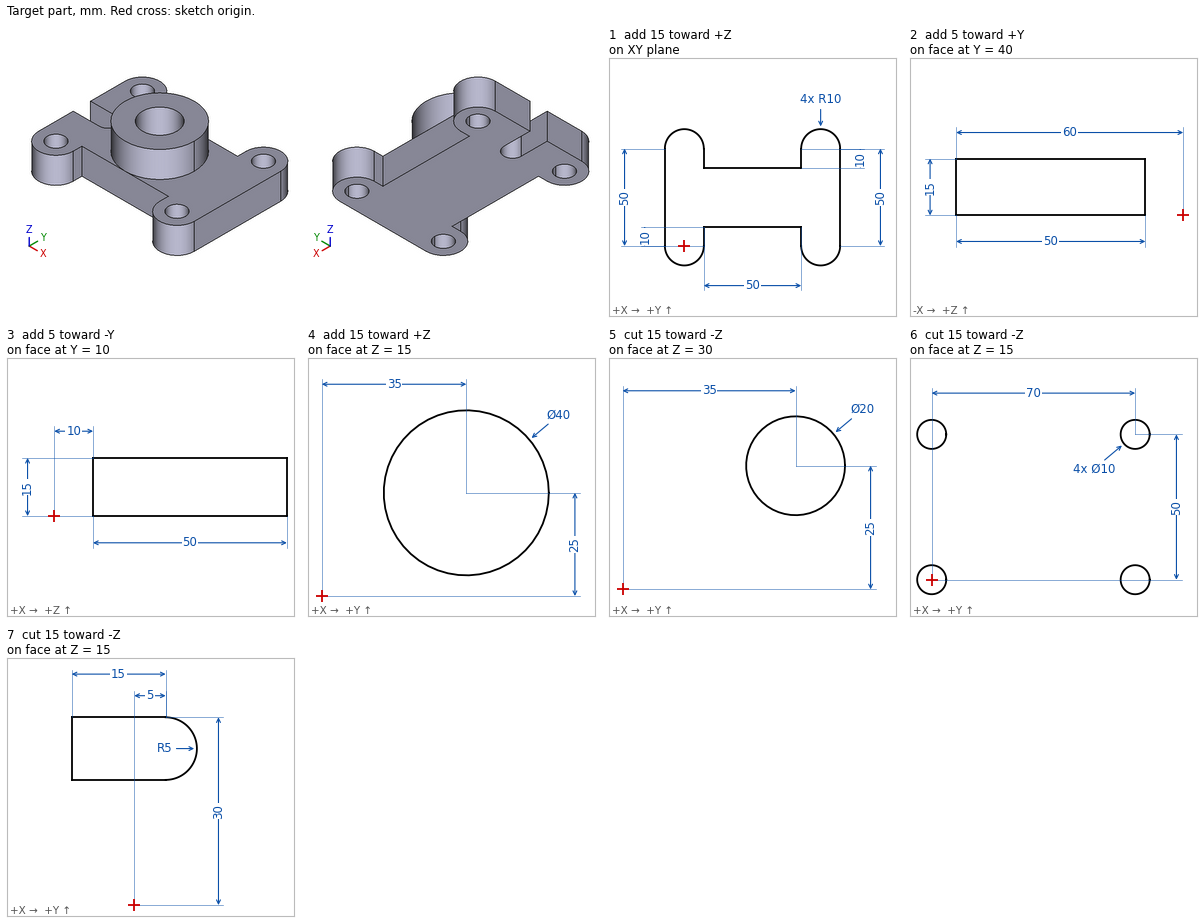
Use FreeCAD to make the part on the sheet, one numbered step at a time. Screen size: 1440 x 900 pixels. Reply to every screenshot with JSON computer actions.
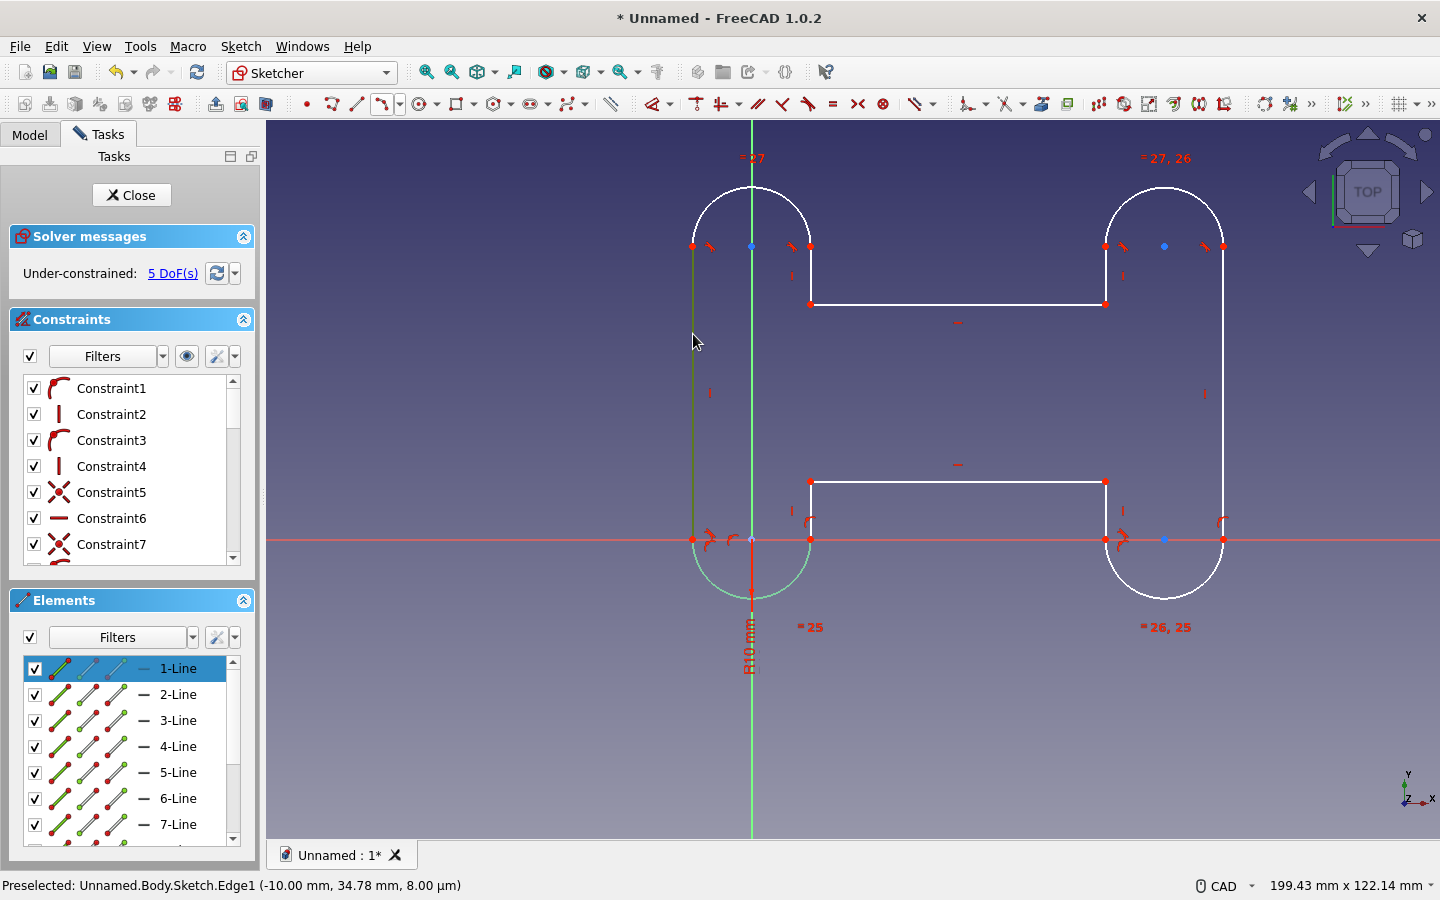
{"action": "key", "text": "i"}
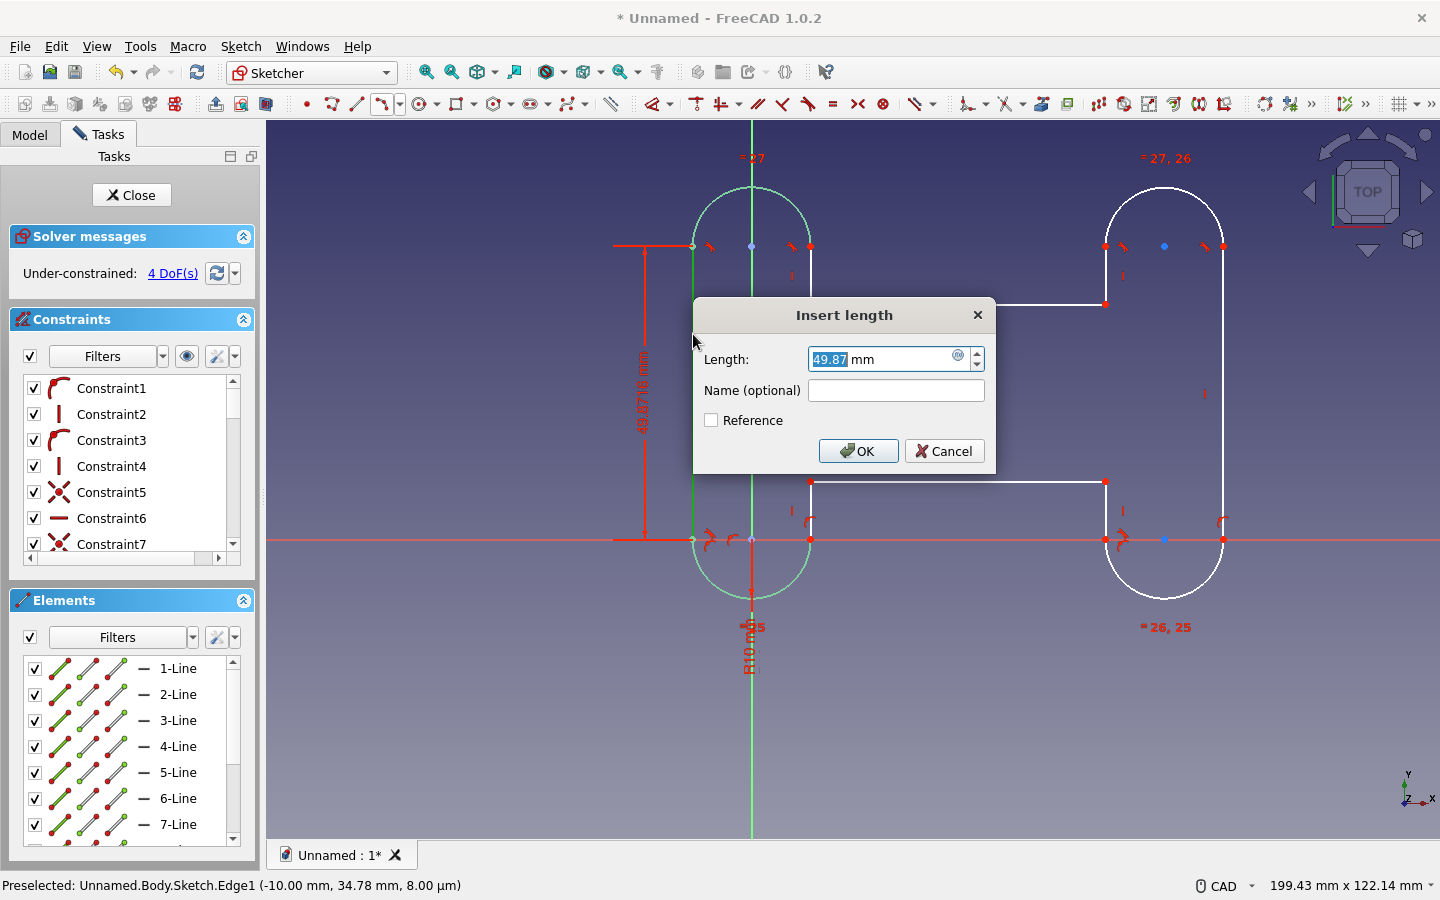
{"action": "type", "text": "50"}
{"action": "key", "text": "Return"}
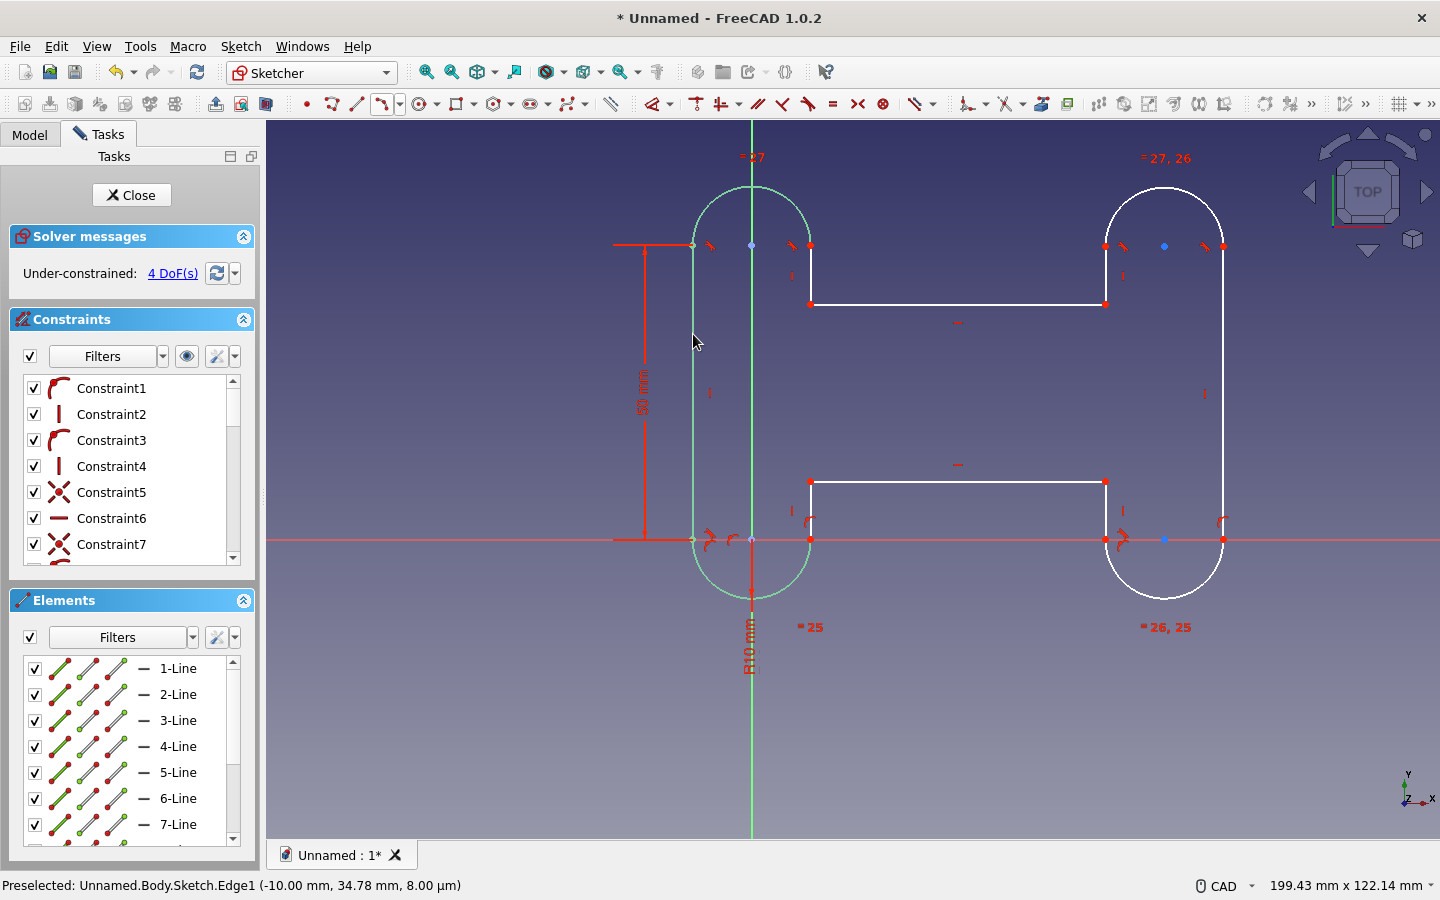
{"action": "left_click", "coordinate": [811, 499]}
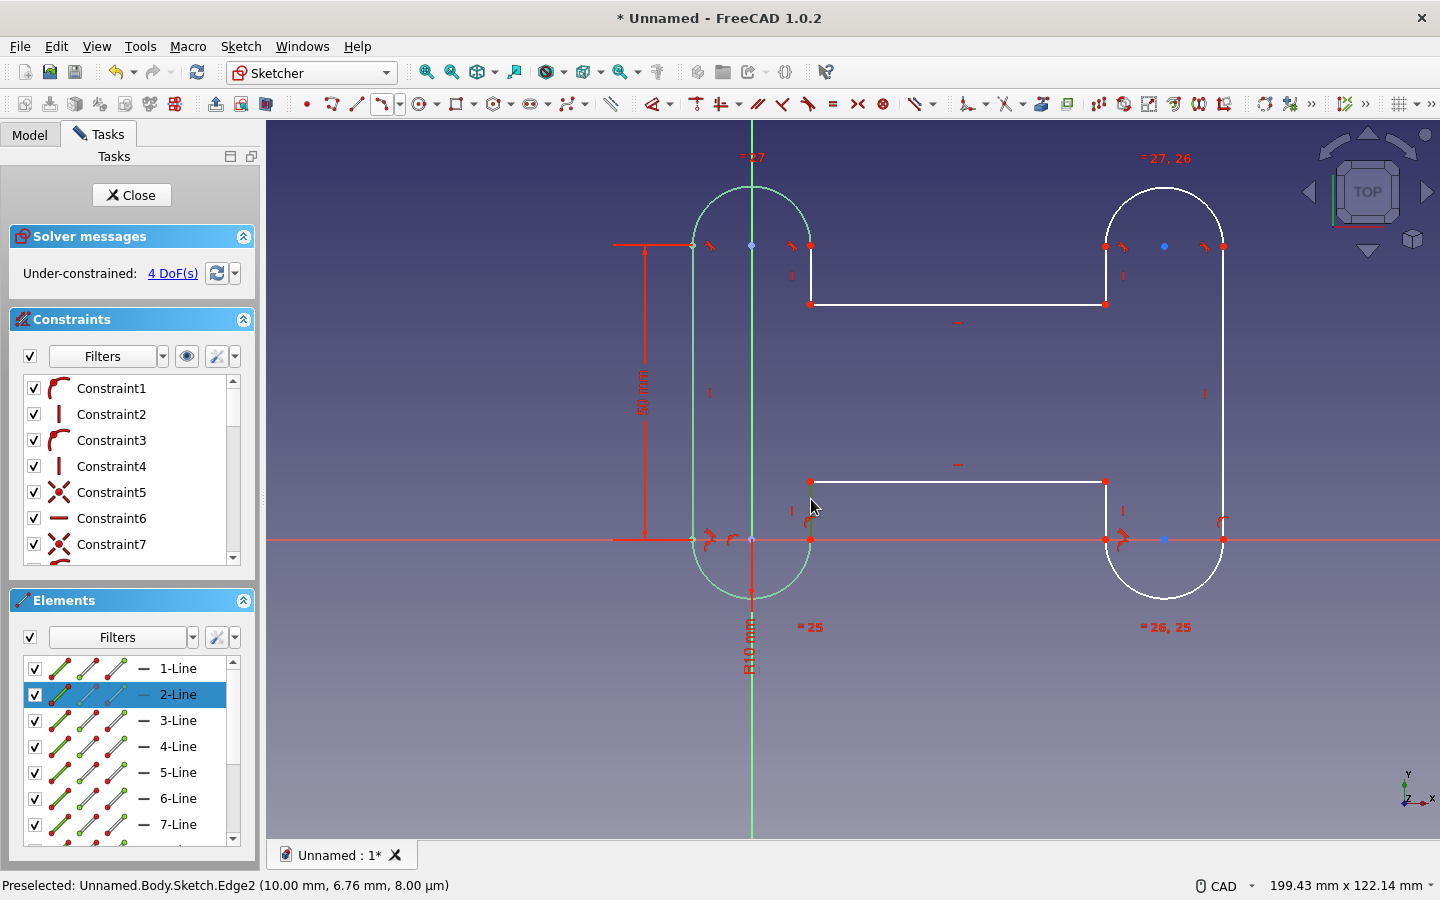
{"action": "key", "text": "i"}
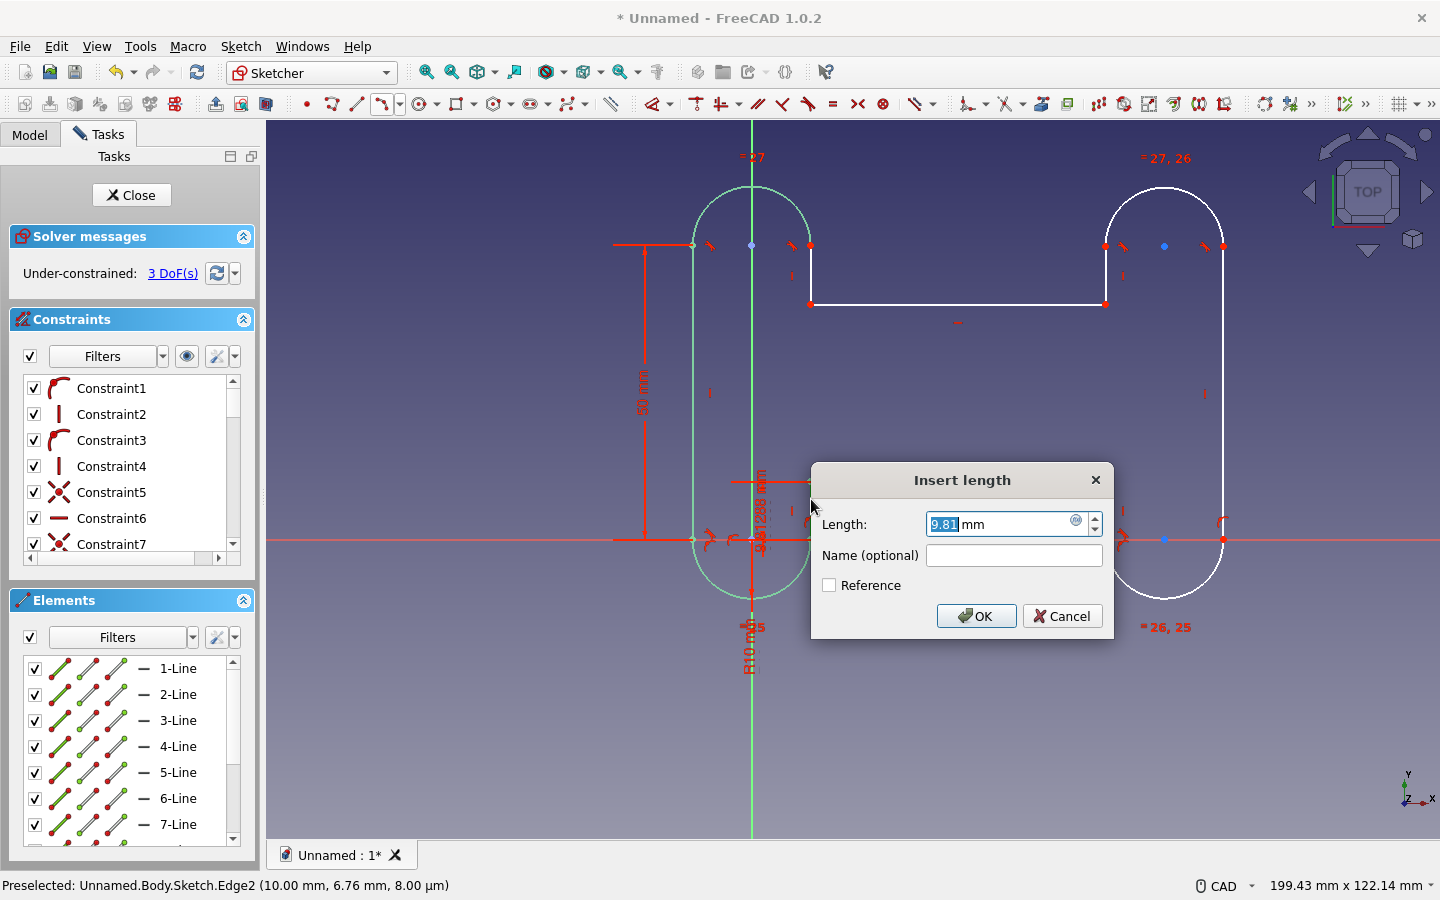
{"action": "type", "text": "10"}
{"action": "key", "text": "Return"}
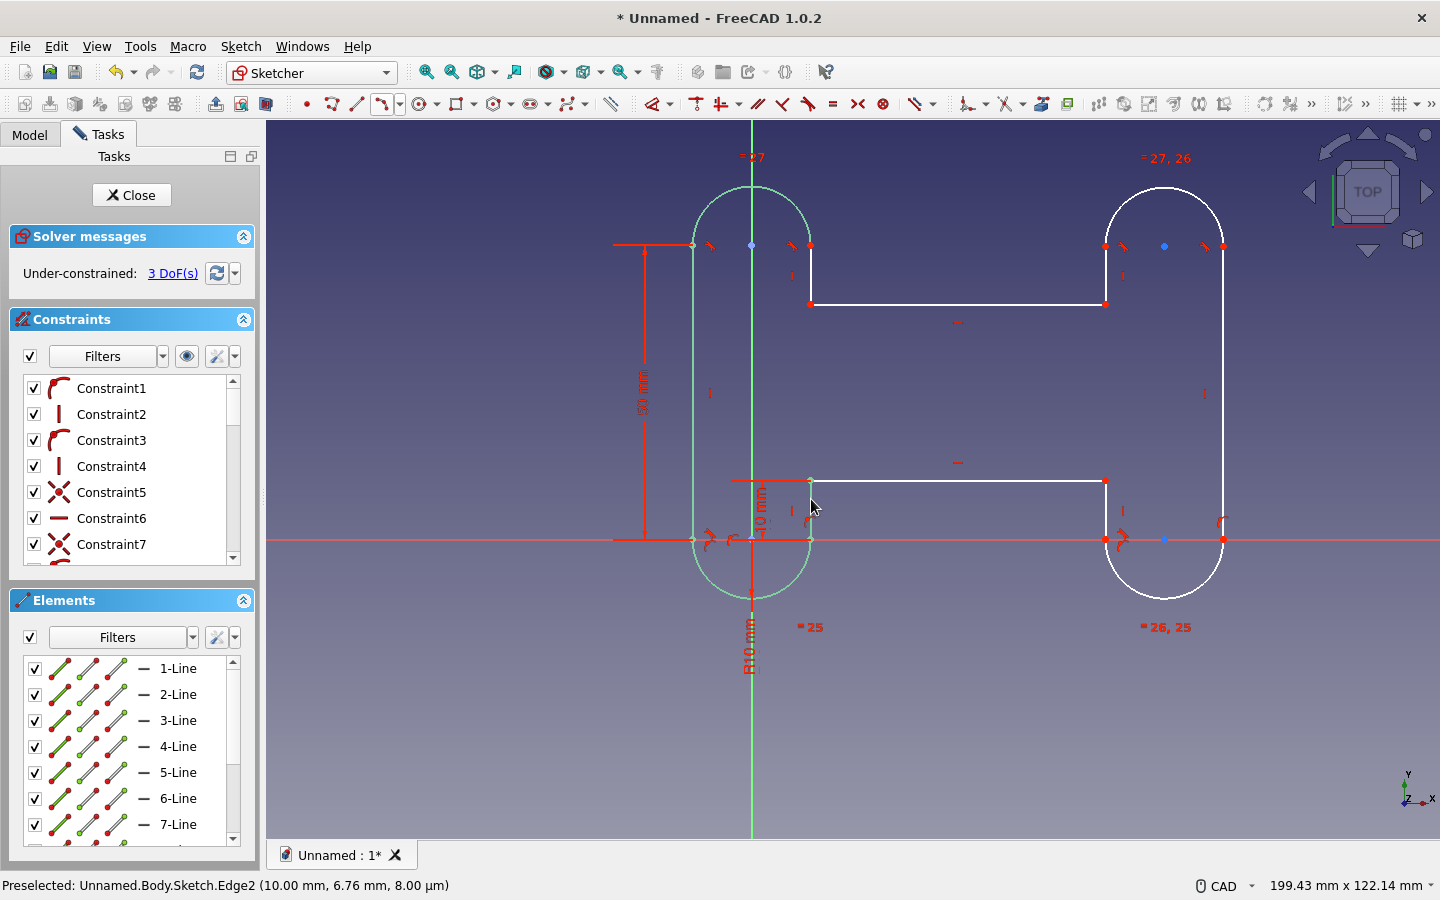
{"action": "left_click", "coordinate": [899, 481]}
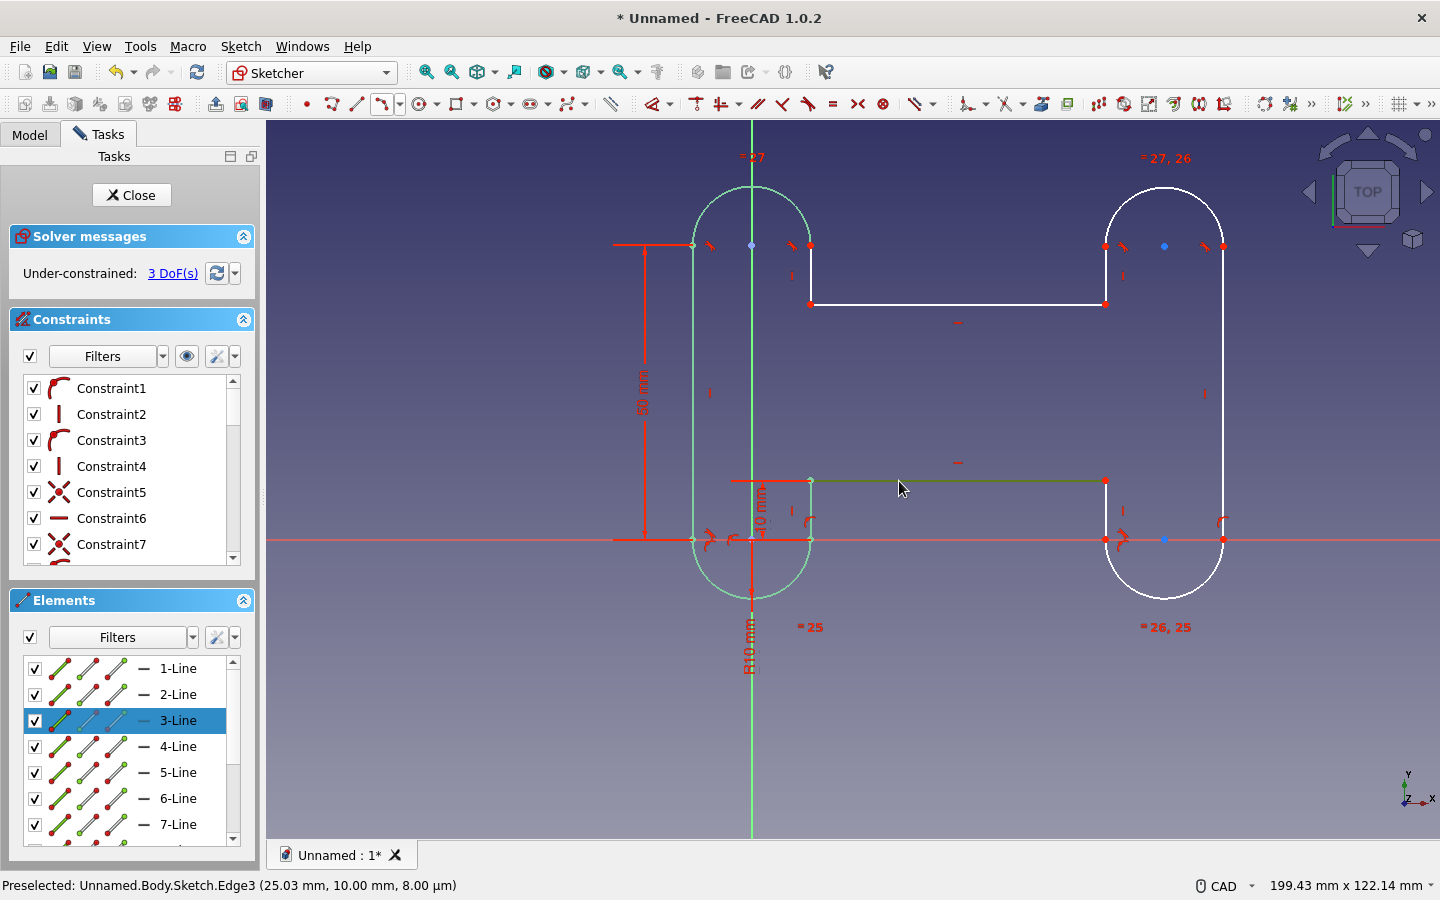
{"action": "left_click", "coordinate": [670, 104]}